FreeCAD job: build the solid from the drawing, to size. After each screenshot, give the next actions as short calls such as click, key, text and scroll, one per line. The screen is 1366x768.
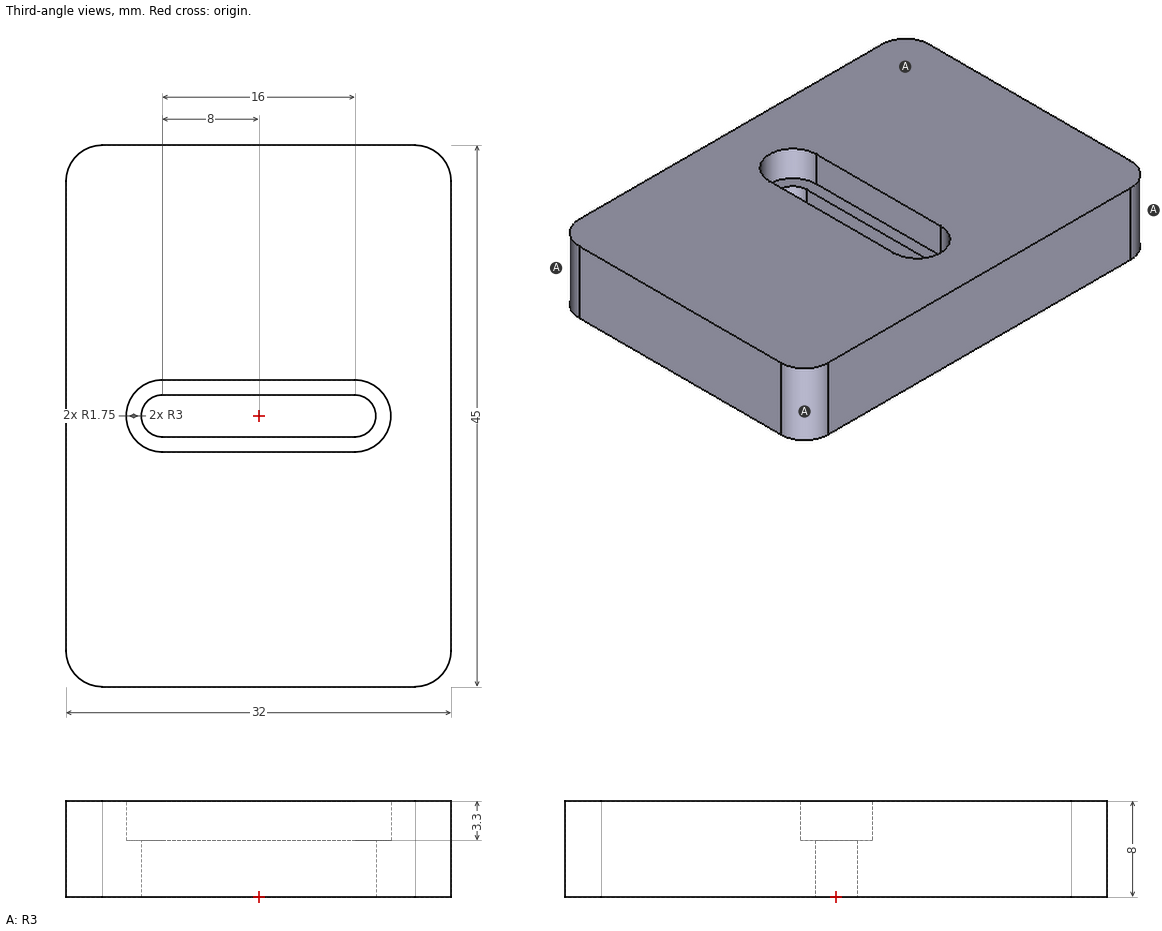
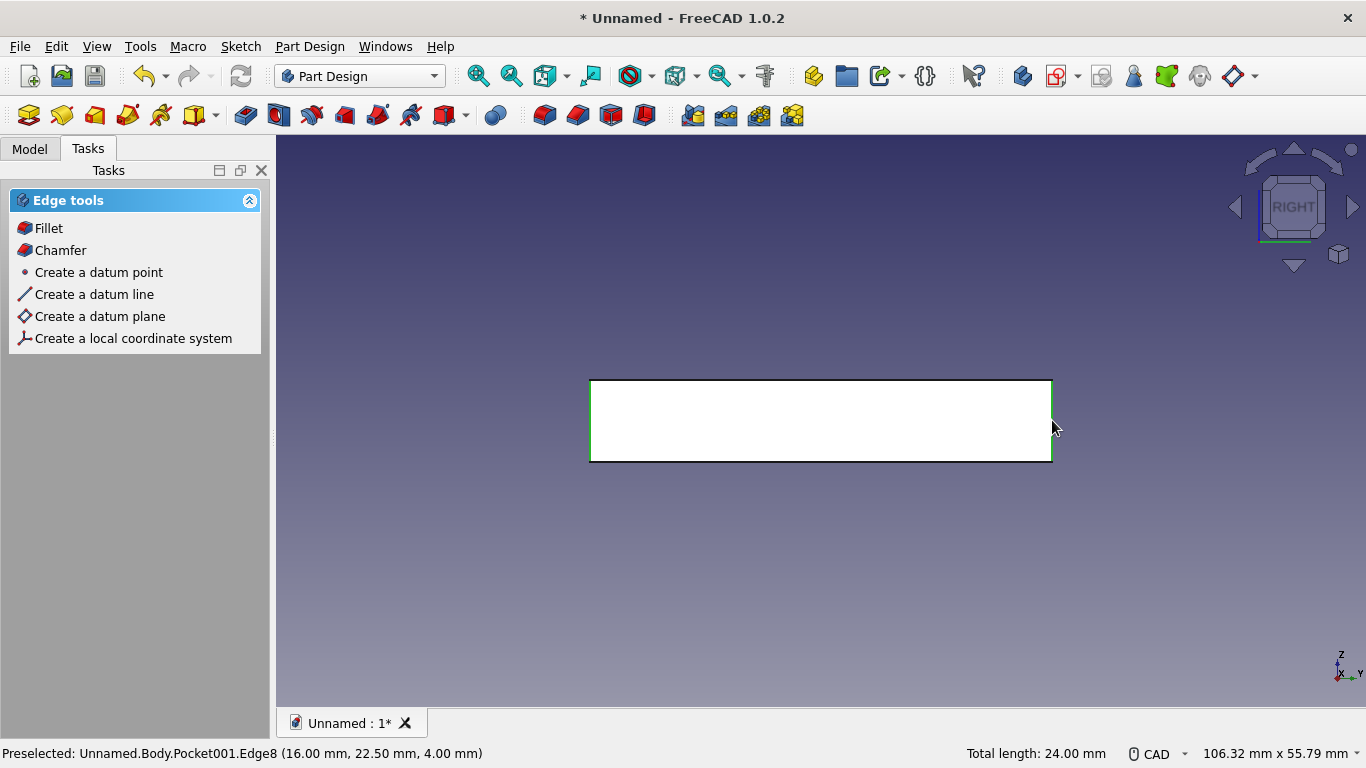
key(5)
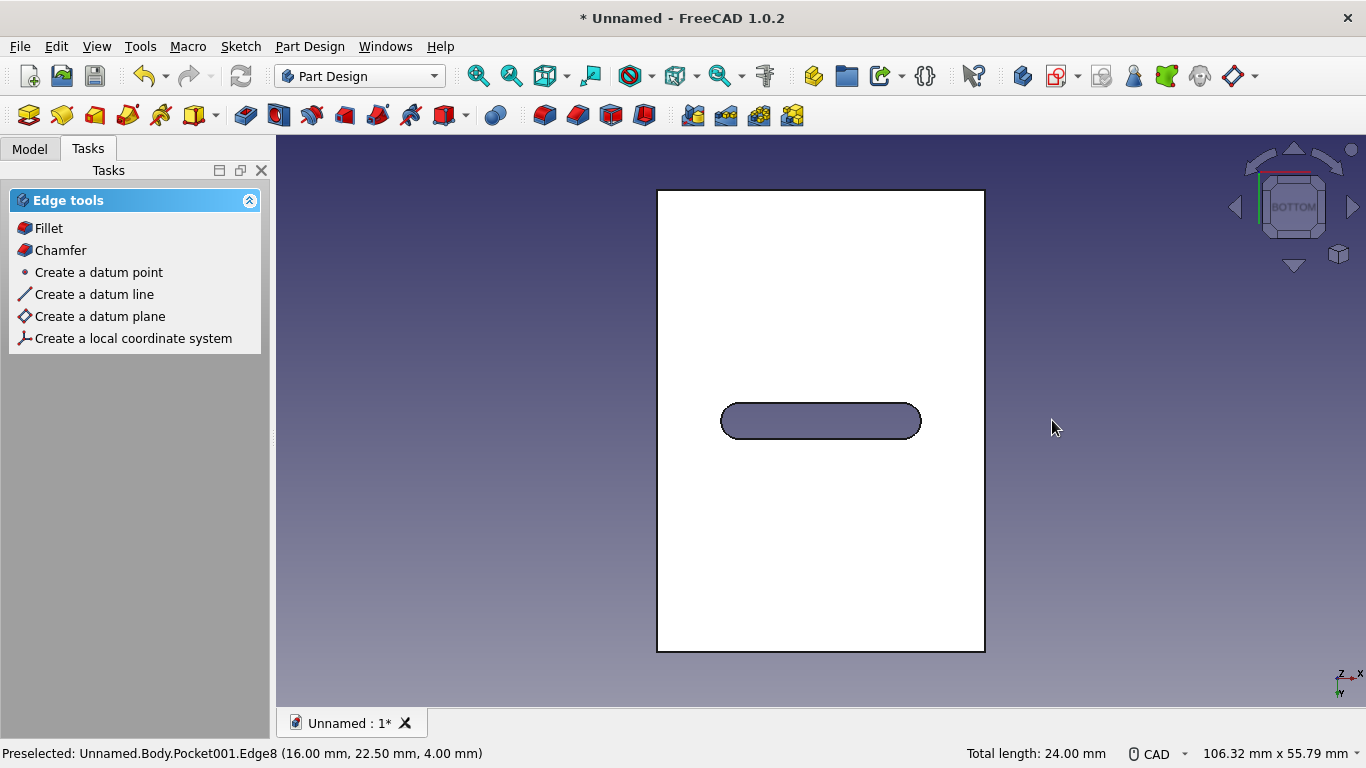
key(4)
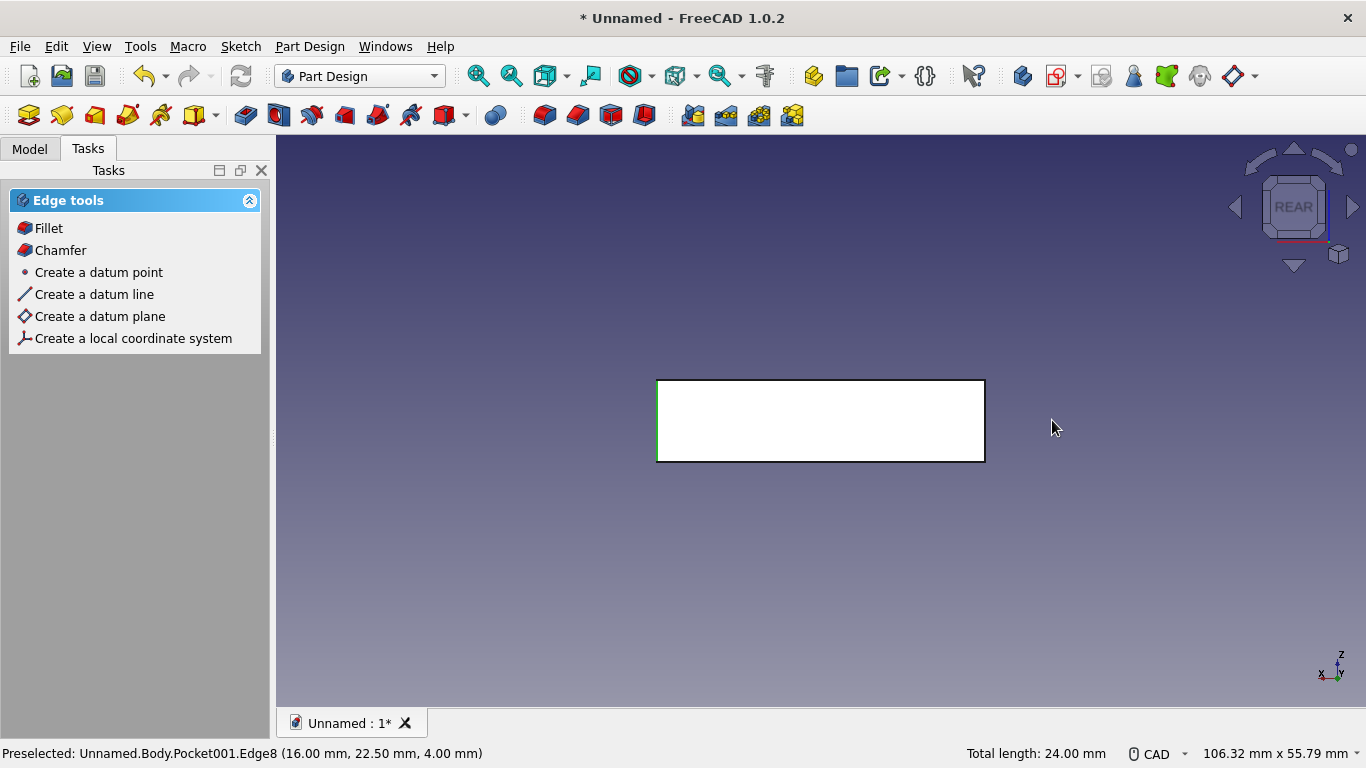
click(479, 76)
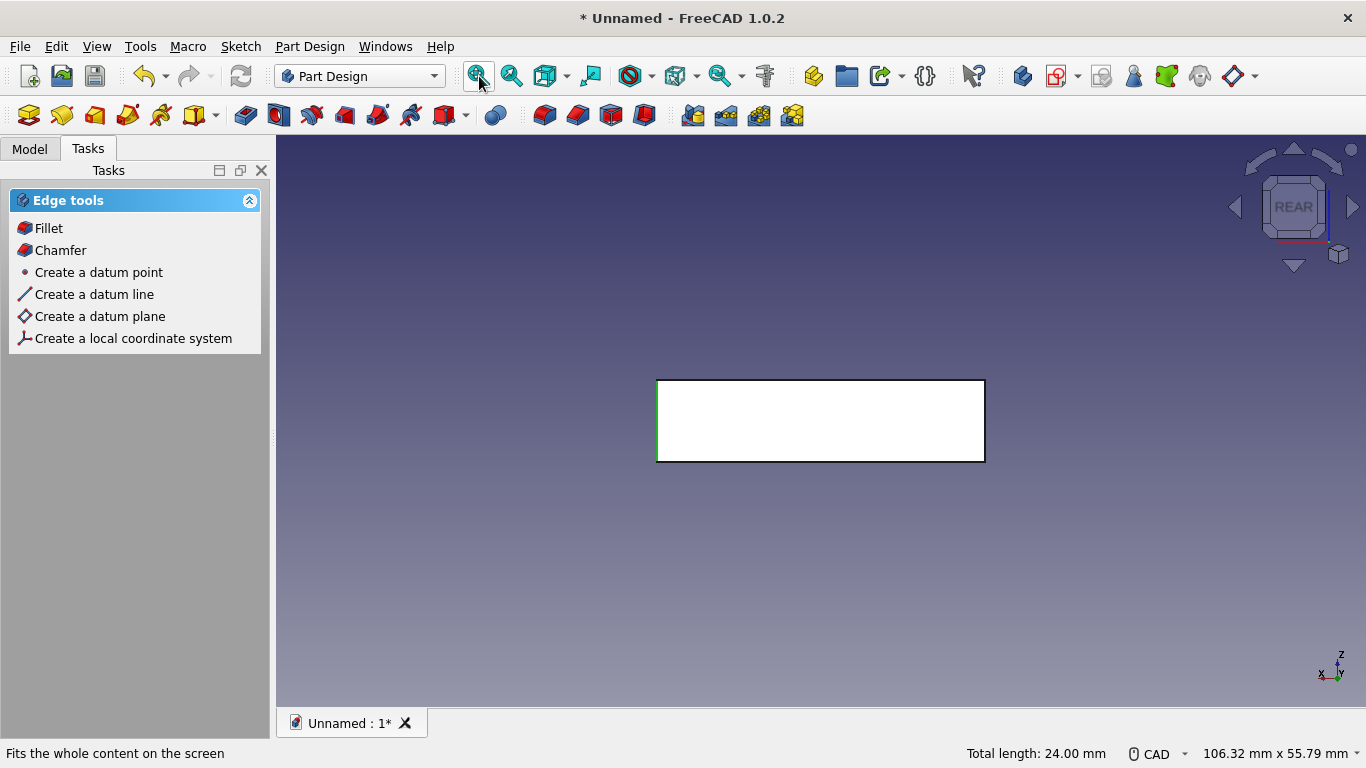
click(985, 420, ctrl)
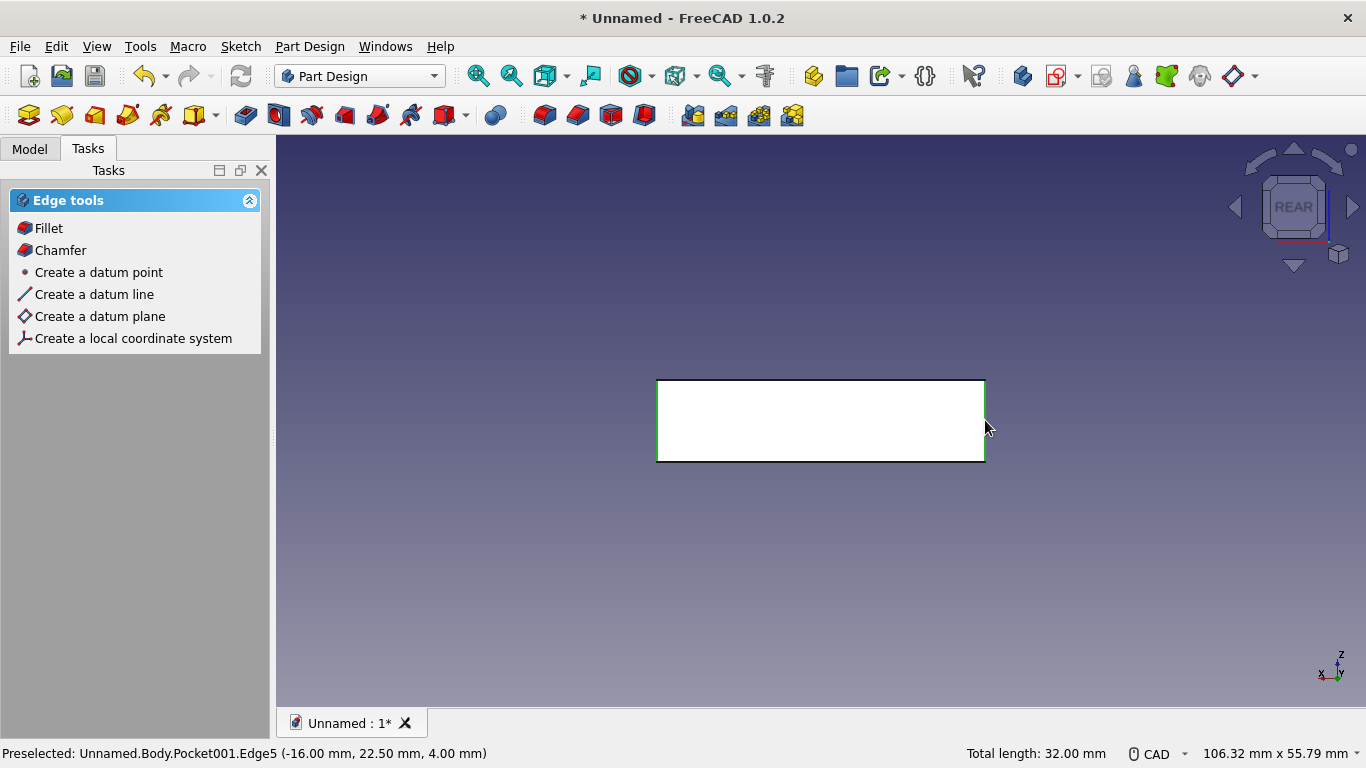
click(545, 116)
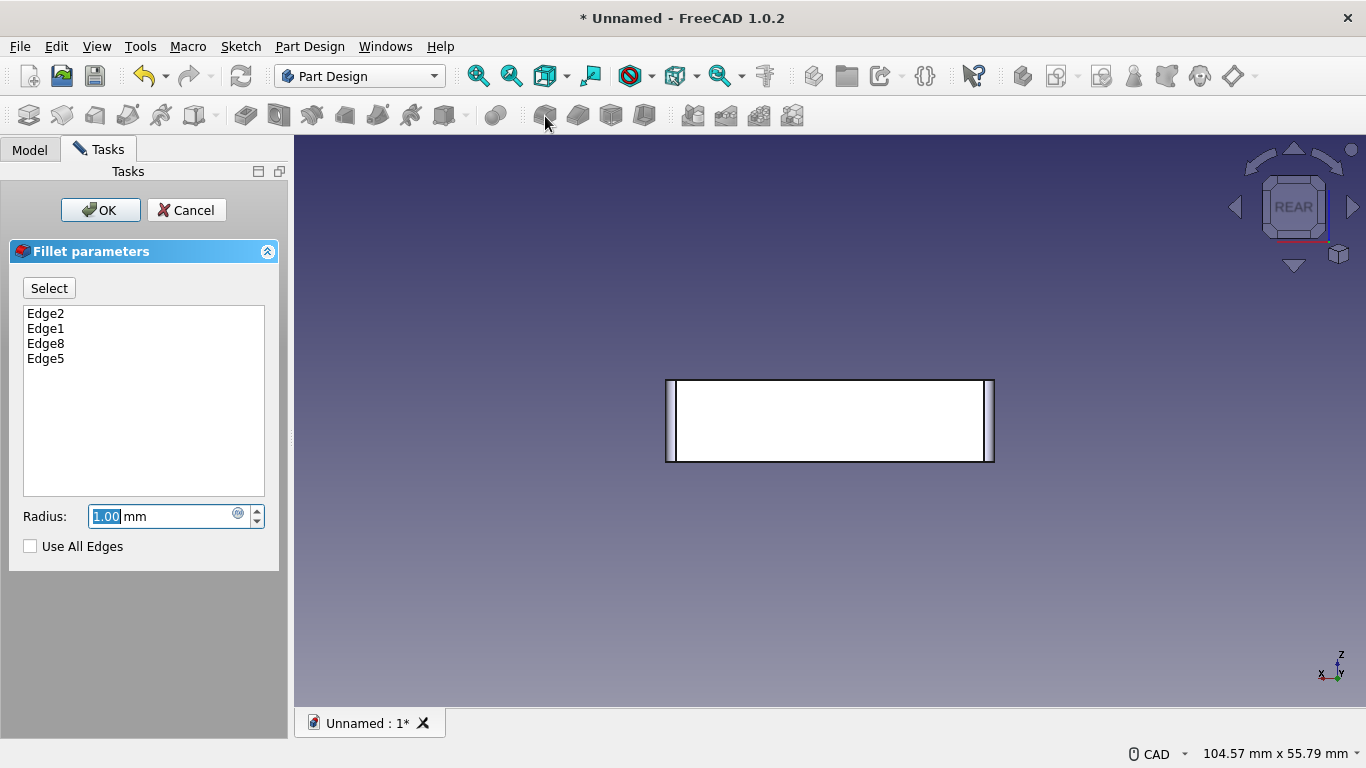
text(3)
key(Tab)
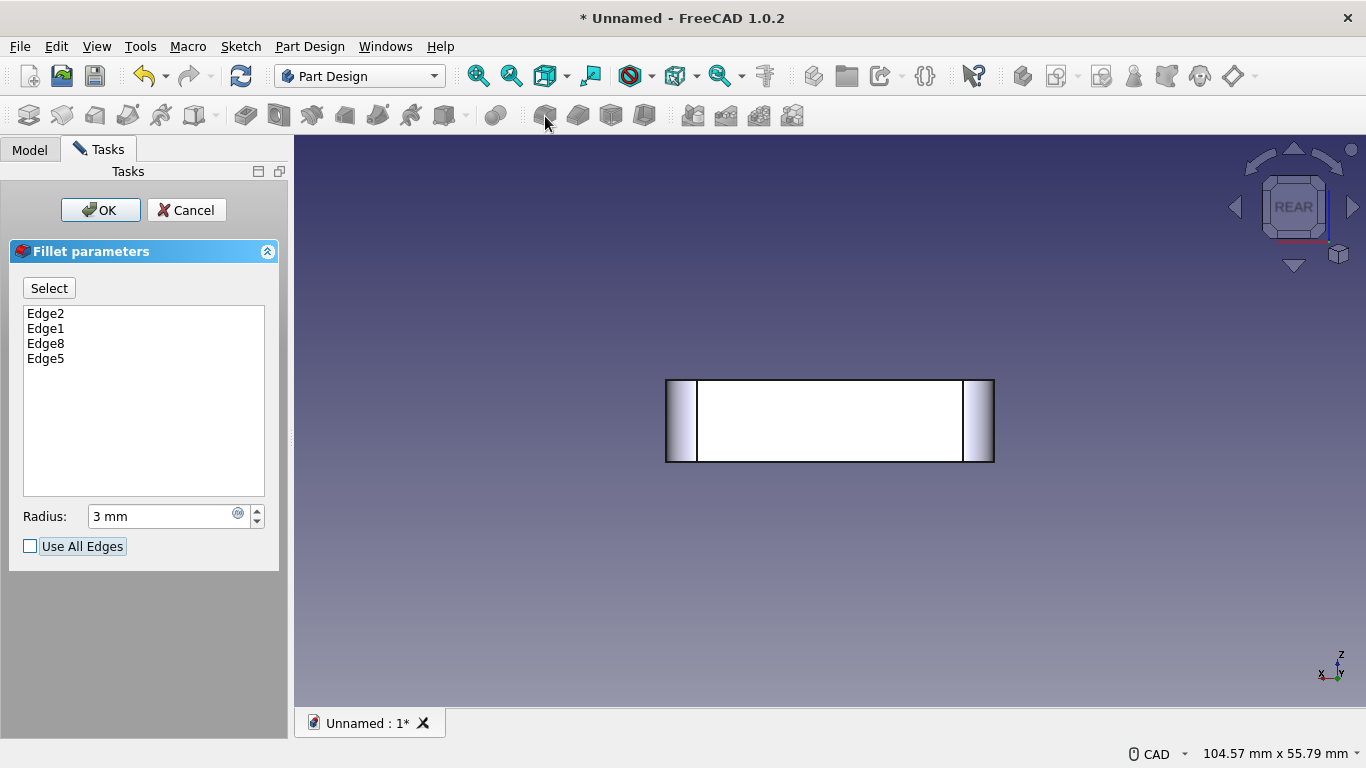
click(101, 210)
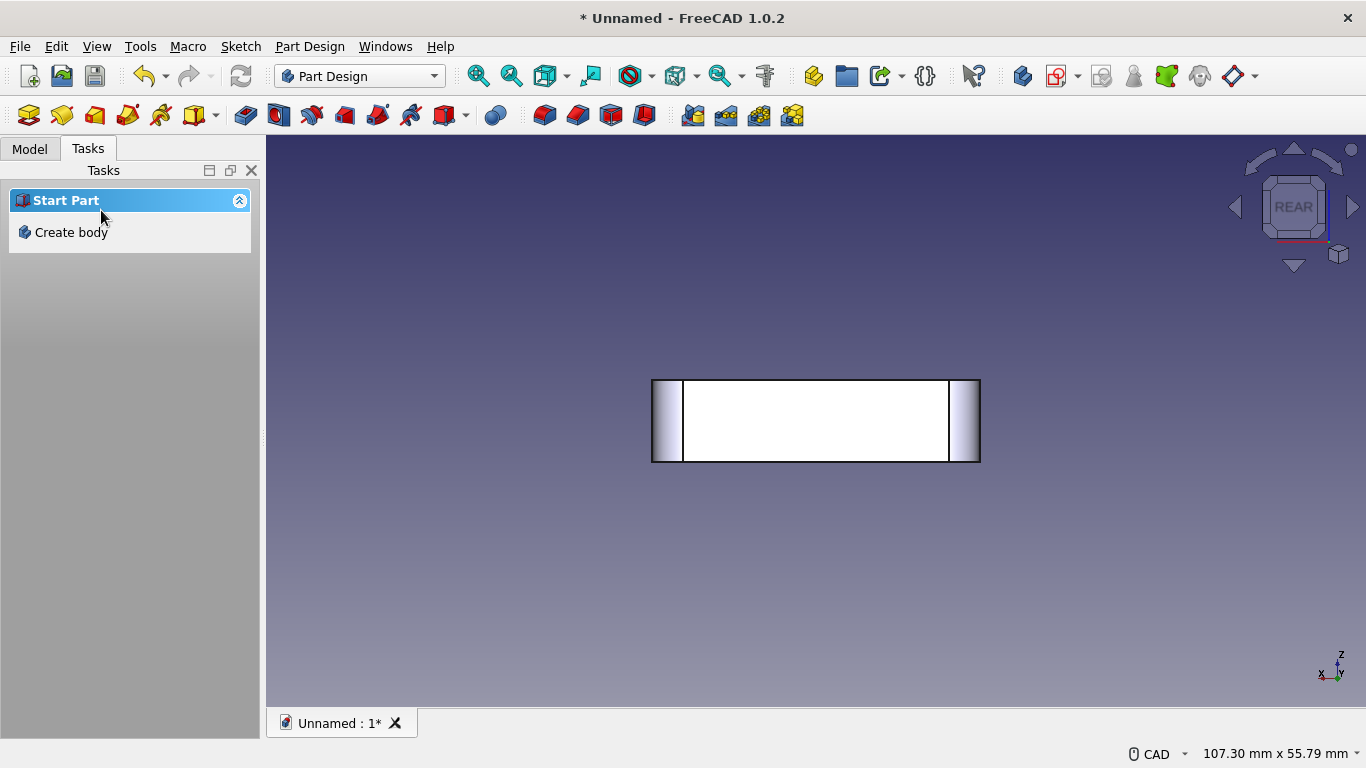
key(0)